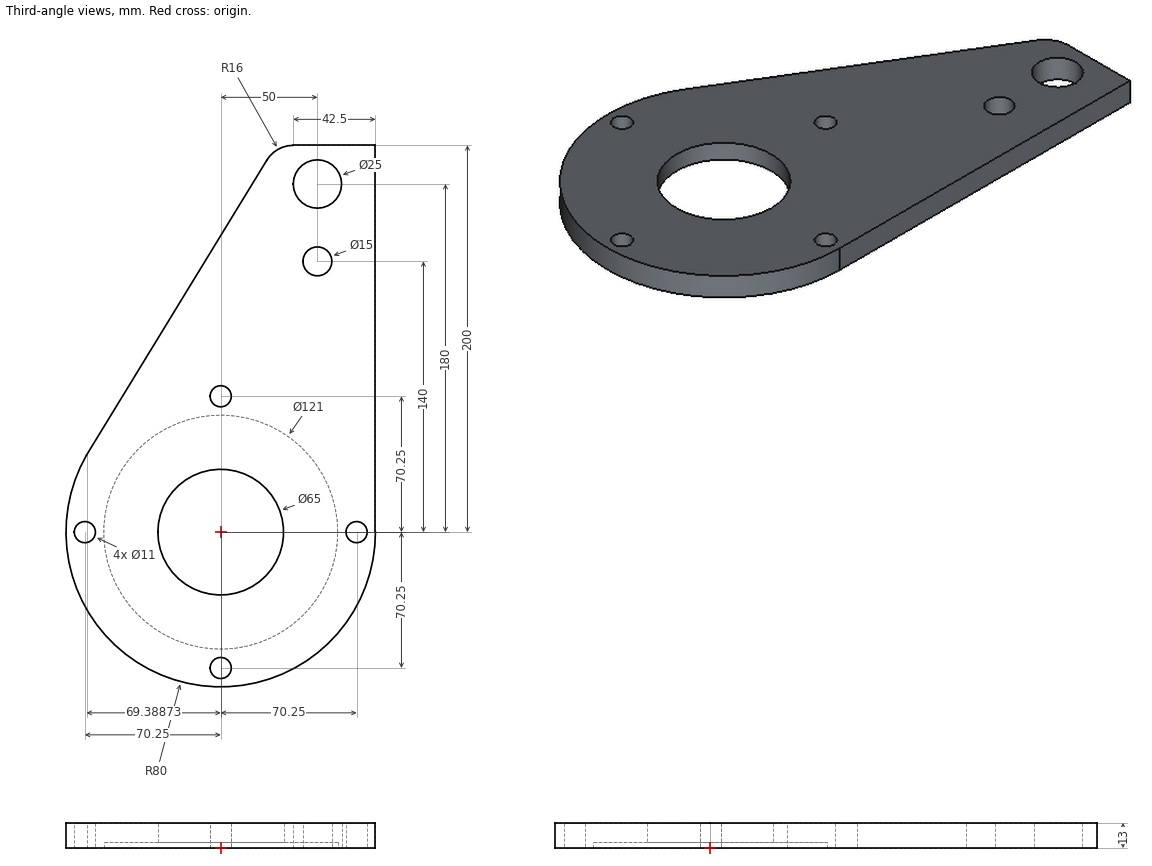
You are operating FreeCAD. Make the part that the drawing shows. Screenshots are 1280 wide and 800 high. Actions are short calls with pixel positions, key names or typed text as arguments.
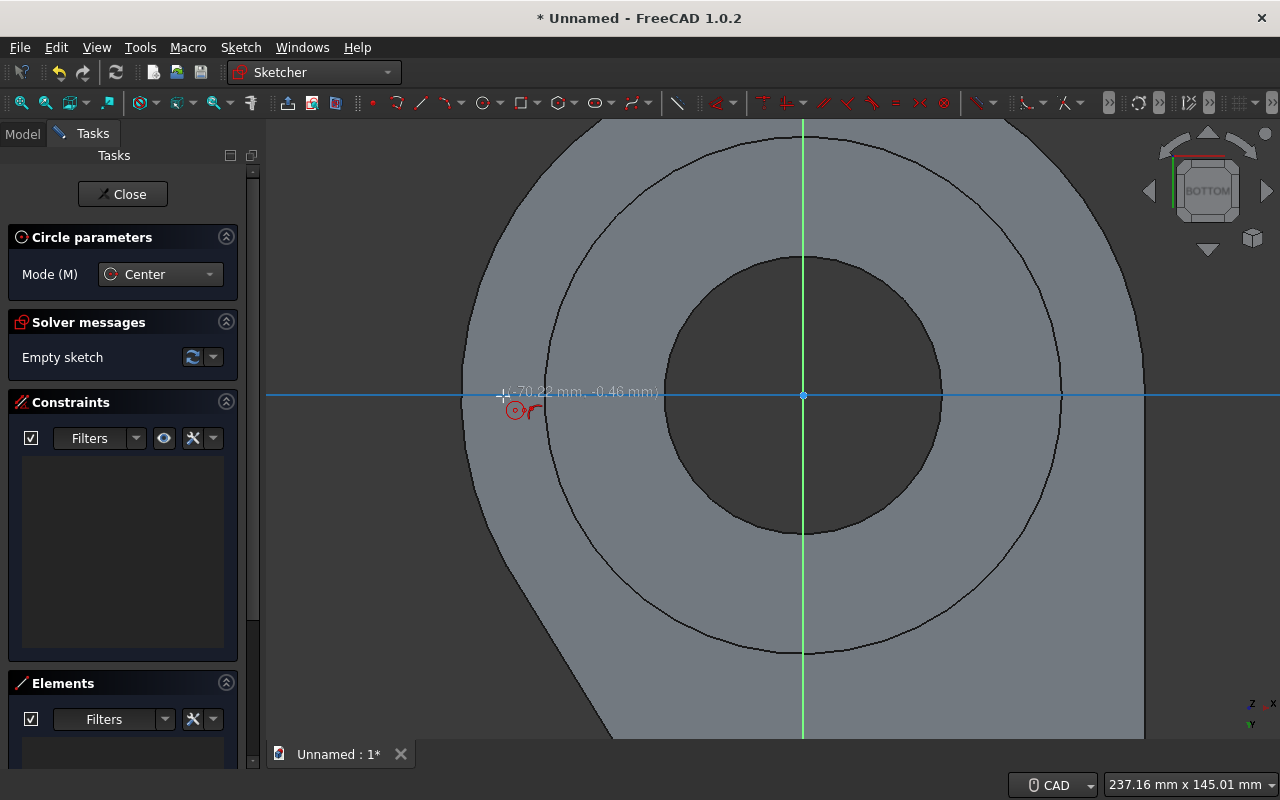
click(503, 395)
click(519, 379)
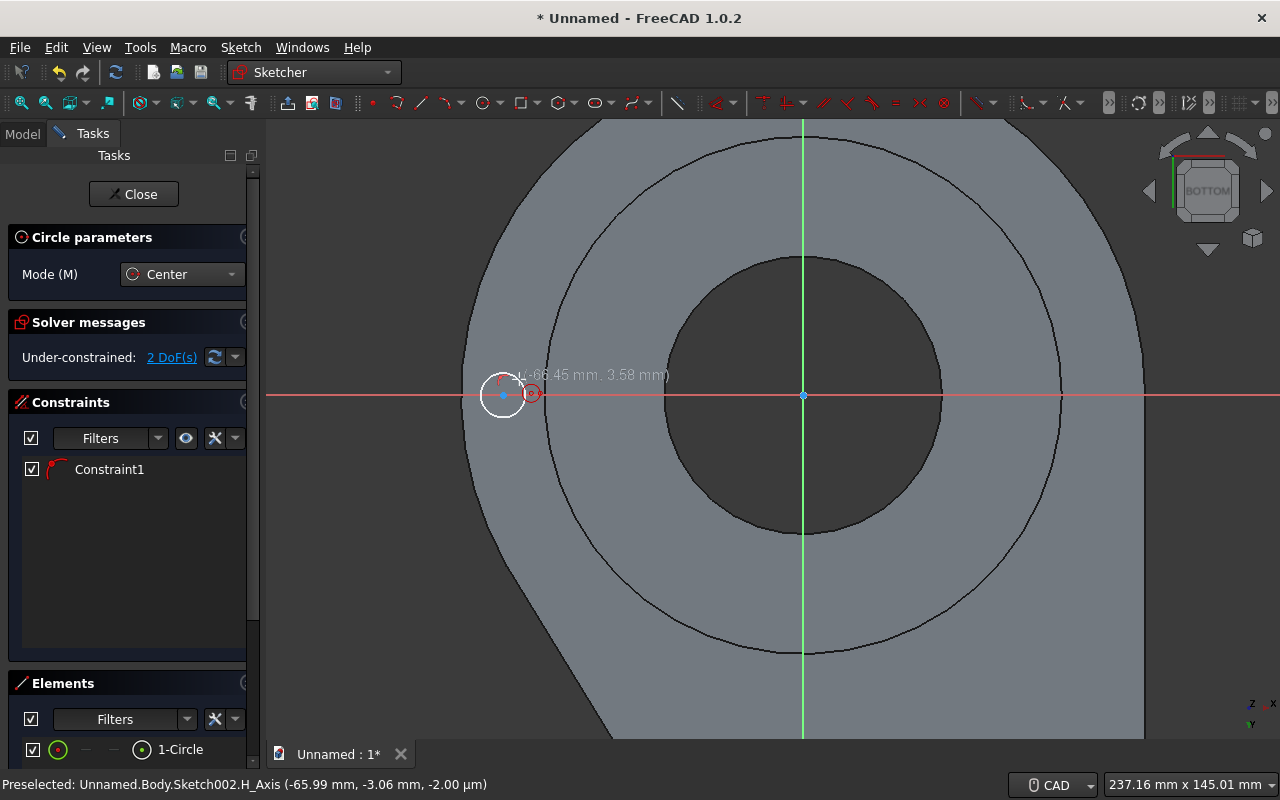
scroll(504, 497, down, 2)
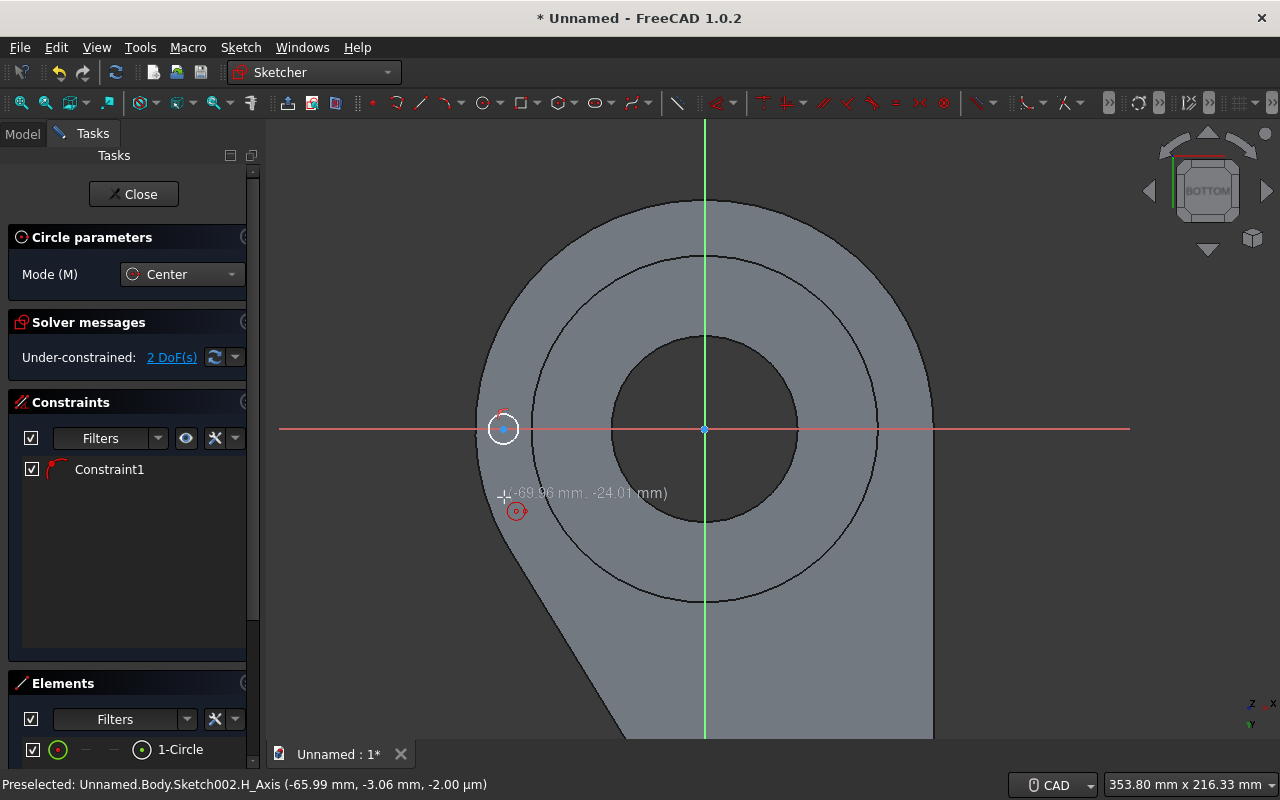
scroll(705, 228, up, 2)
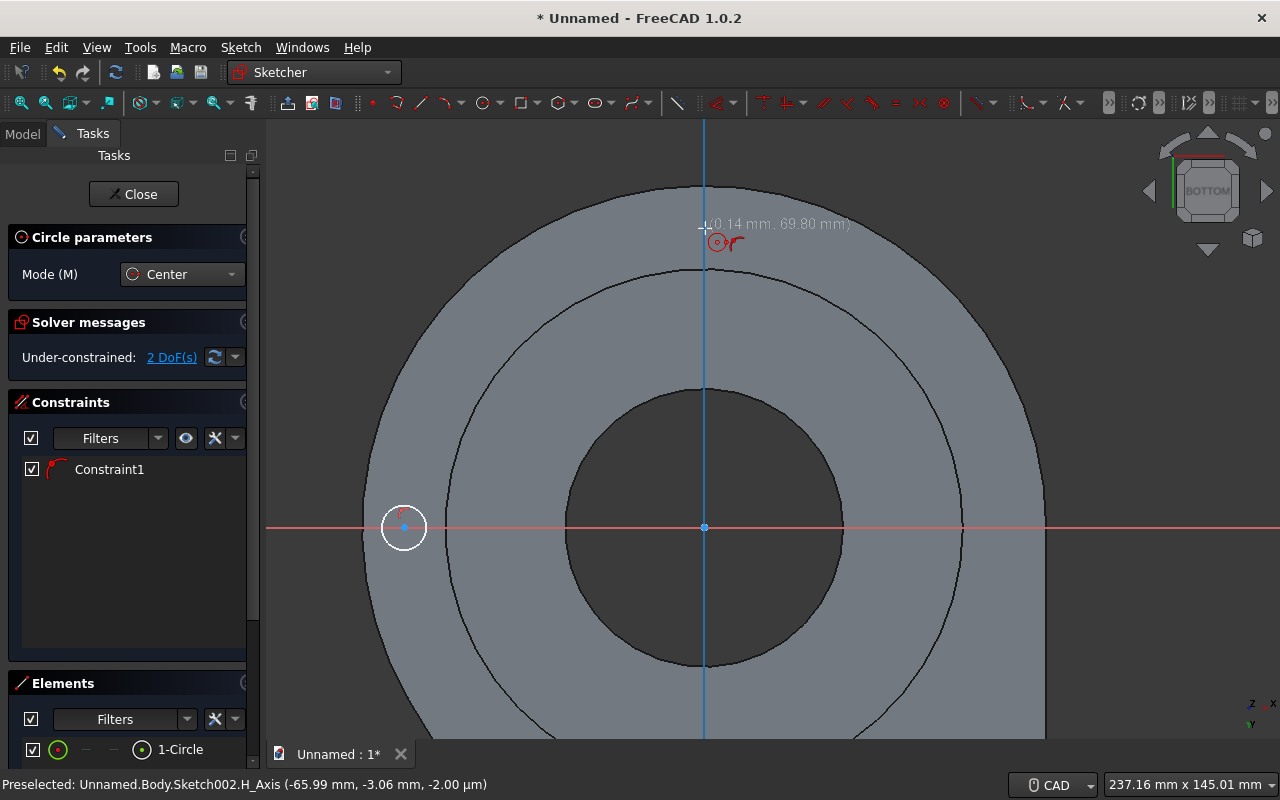
click(704, 227)
click(721, 211)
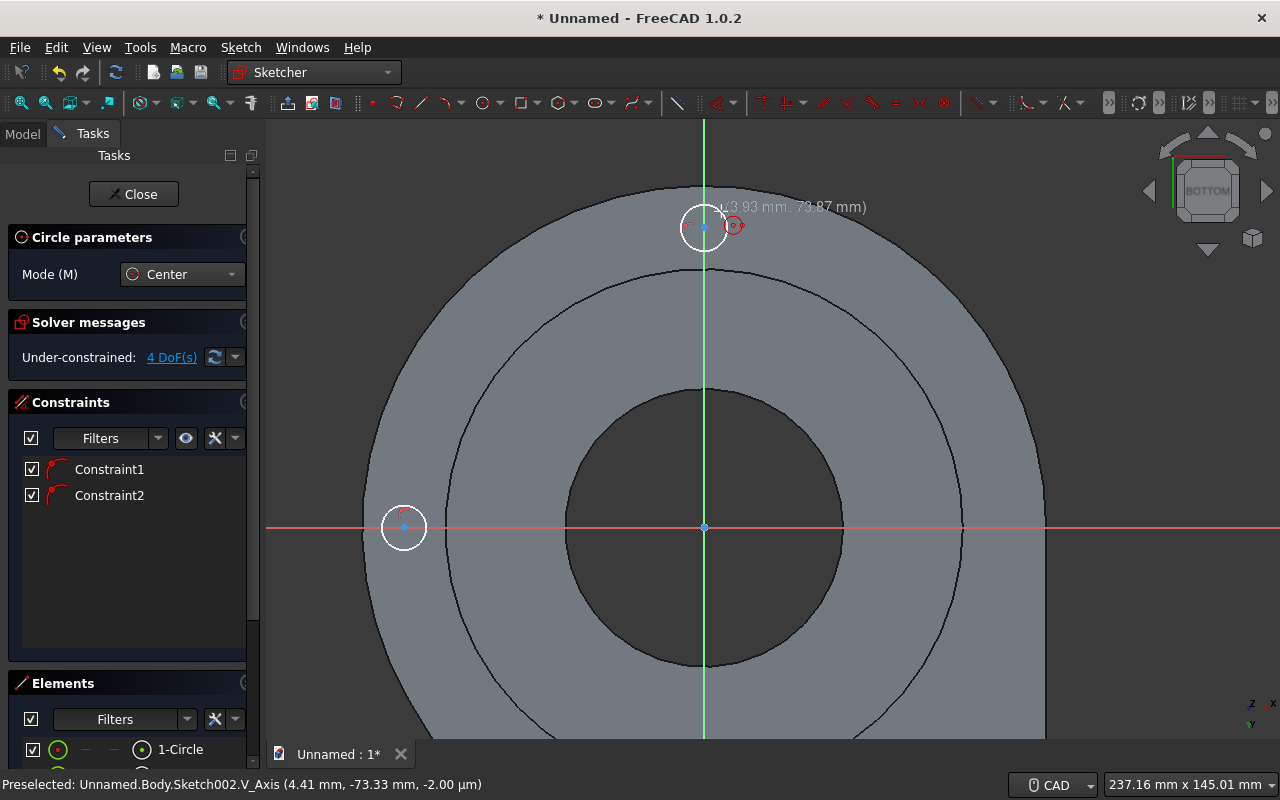
click(1005, 528)
click(1021, 511)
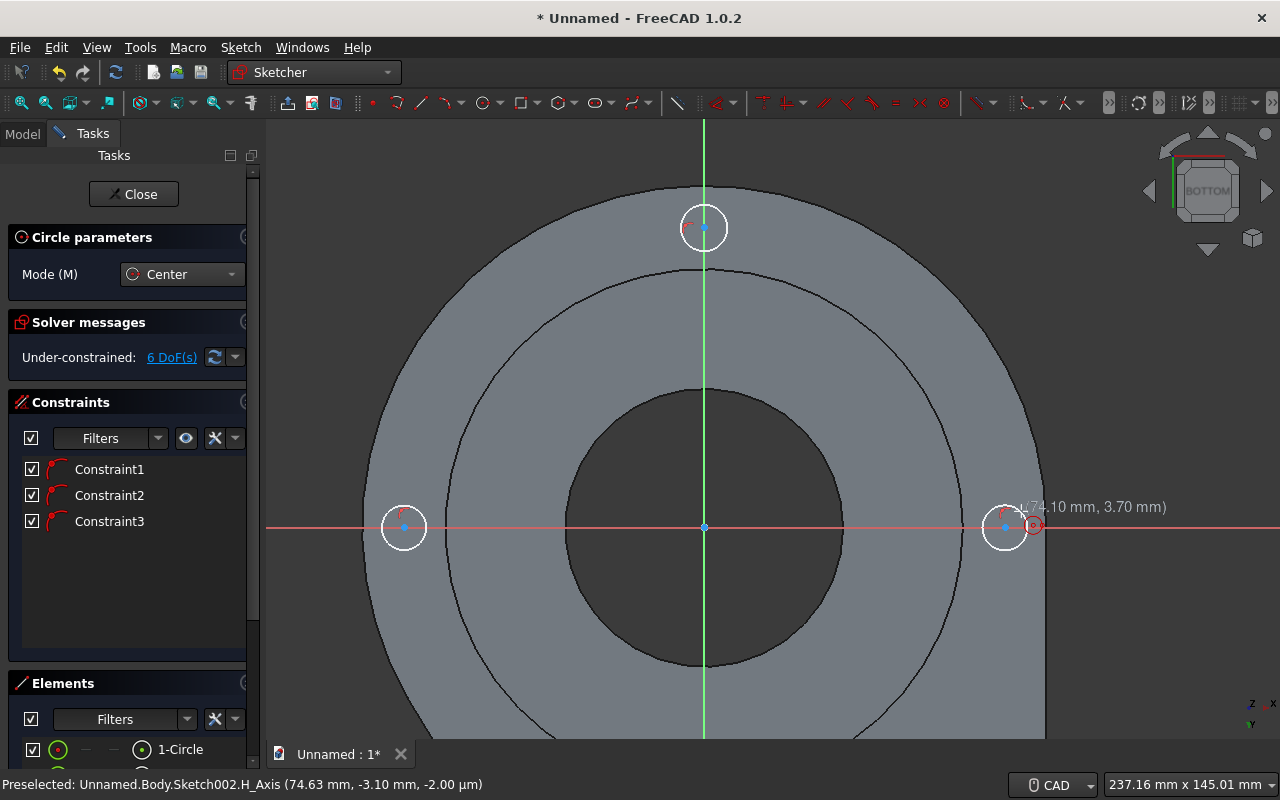
scroll(705, 228, down, 2)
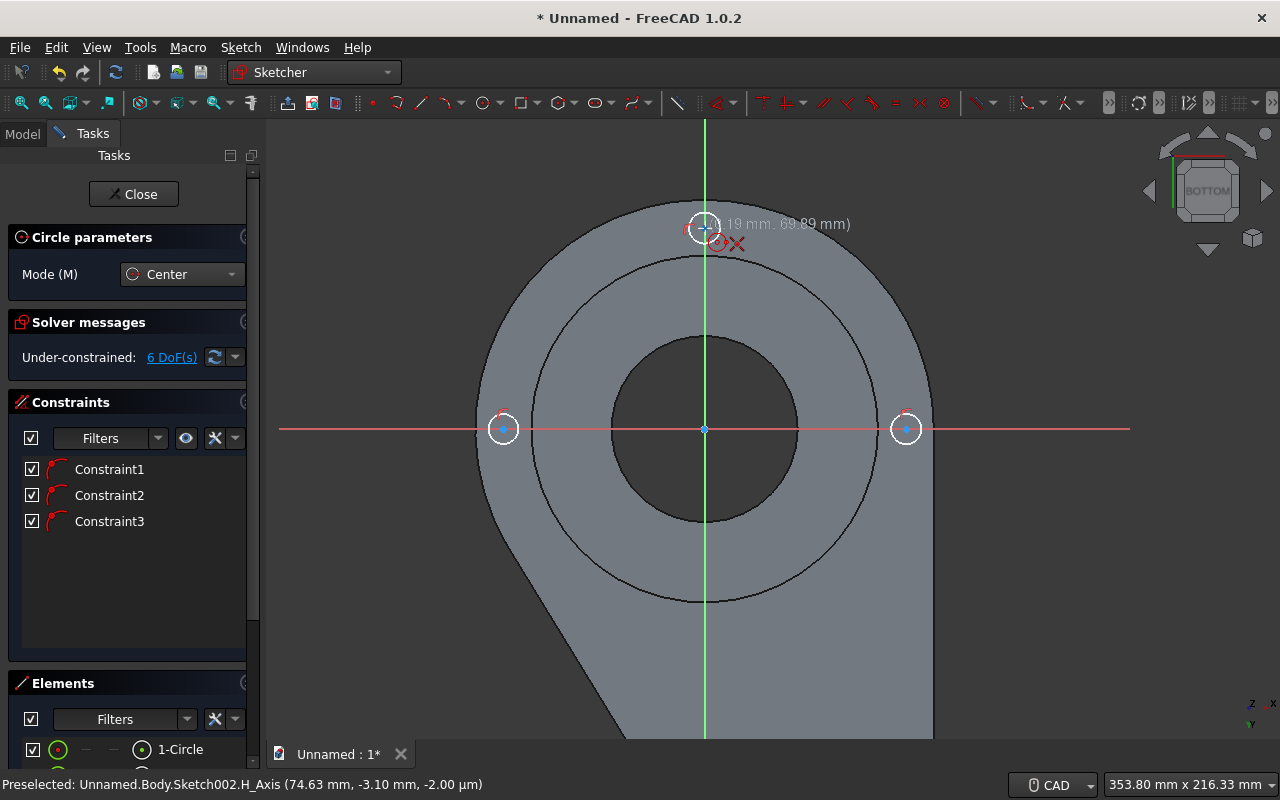
scroll(705, 630, up, 2)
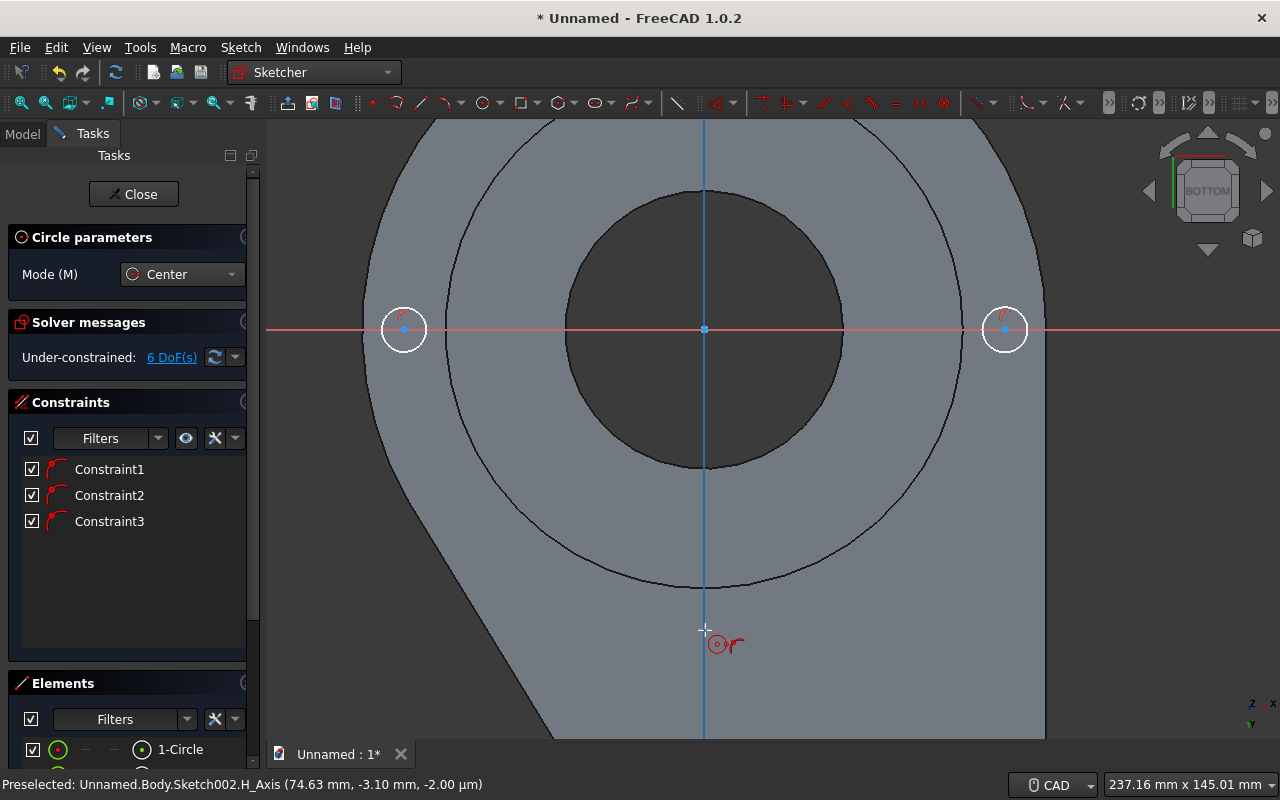
click(704, 630)
click(721, 614)
key(Escape)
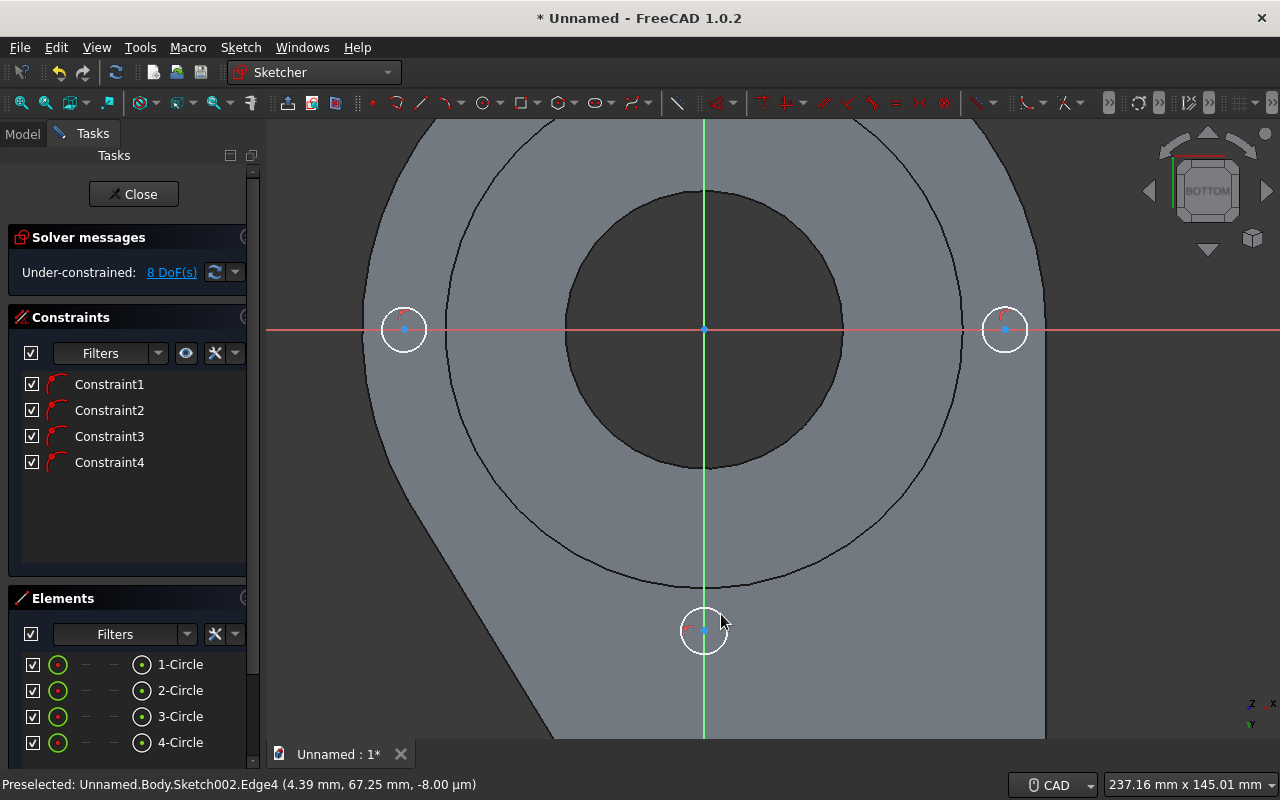
click(420, 314)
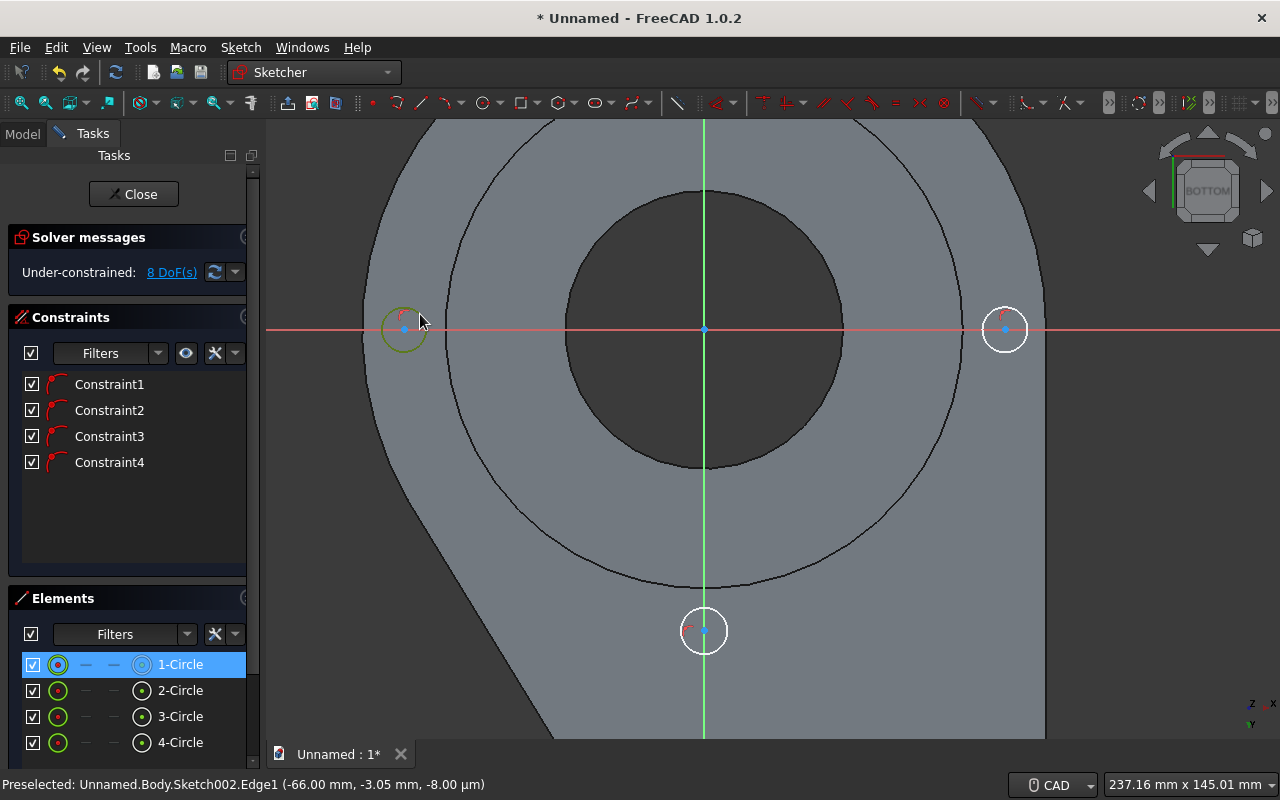
scroll(705, 631, down, 2)